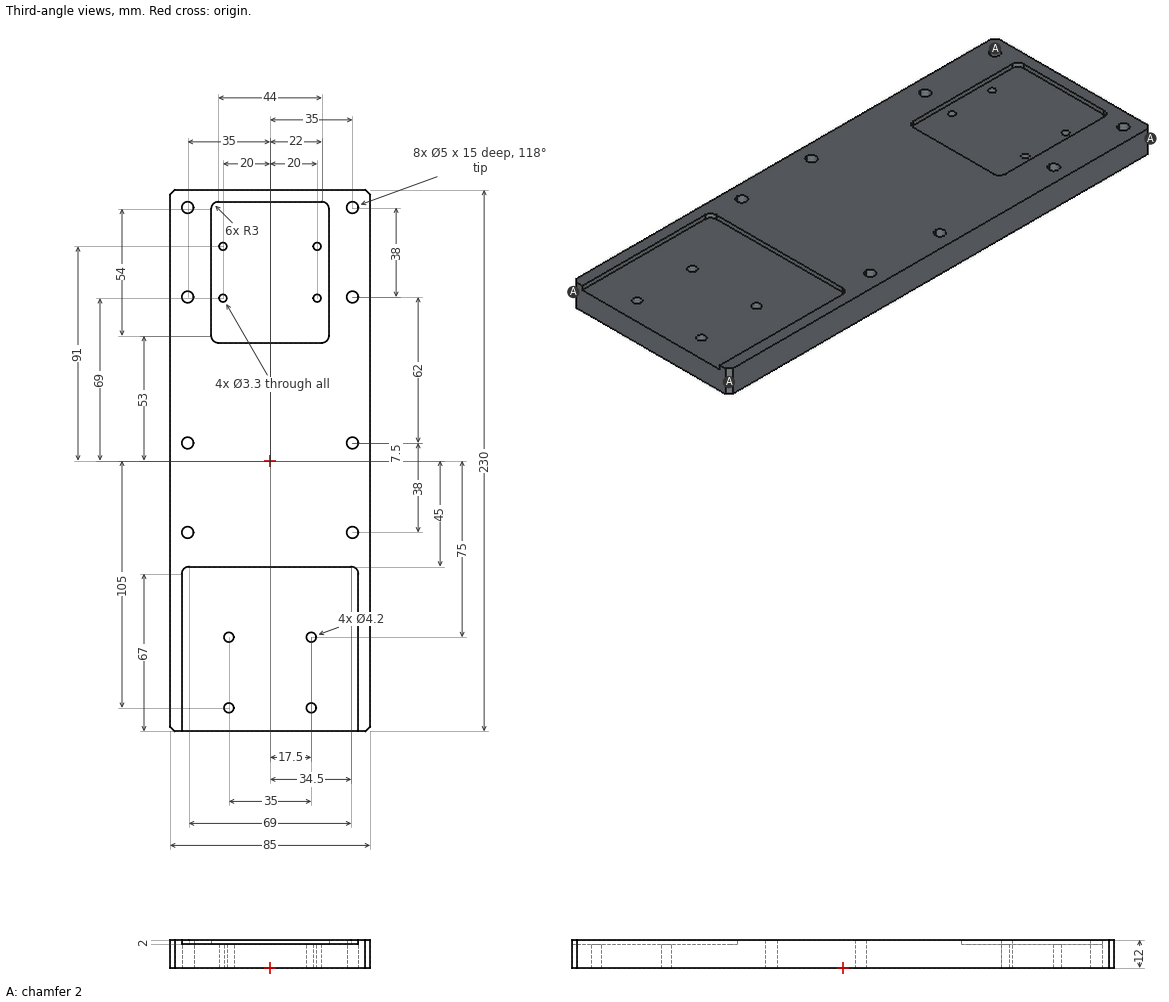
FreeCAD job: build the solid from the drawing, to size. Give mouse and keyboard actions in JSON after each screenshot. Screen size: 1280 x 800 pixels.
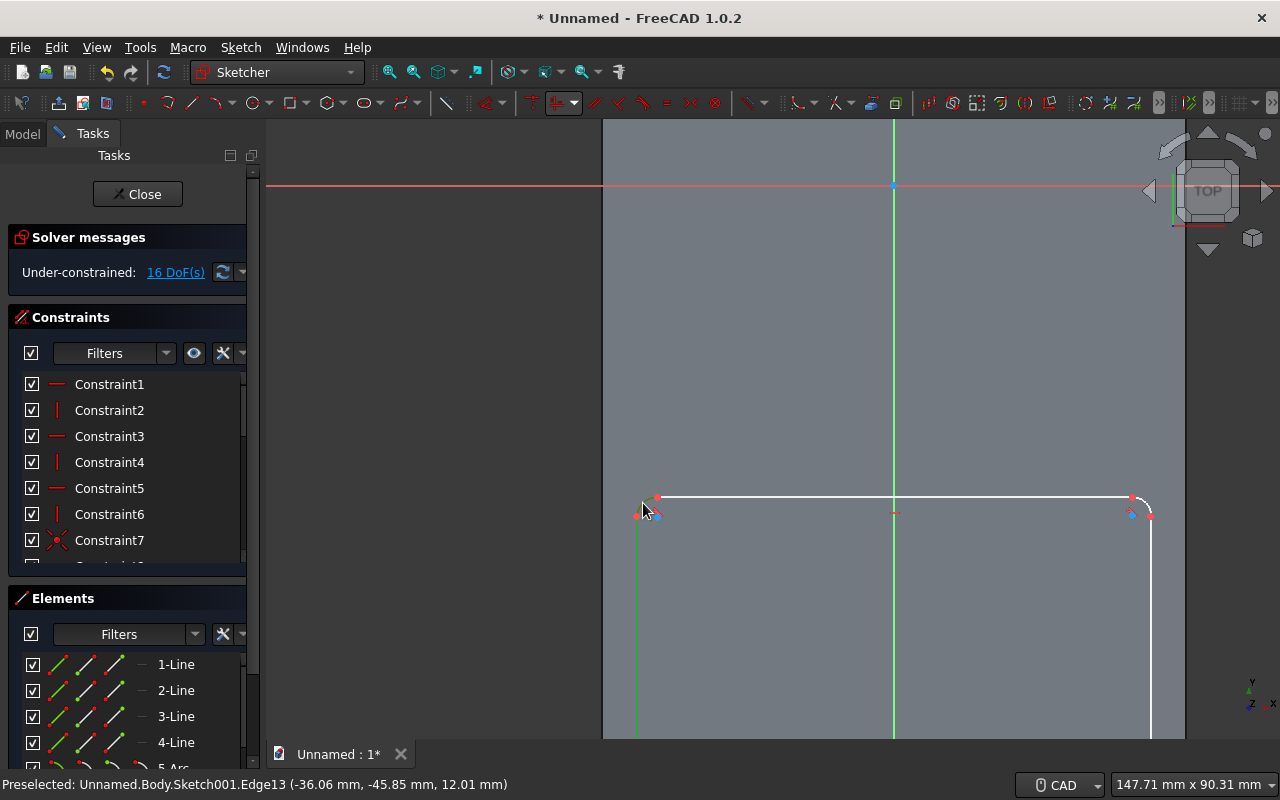
{"action": "key", "text": "t"}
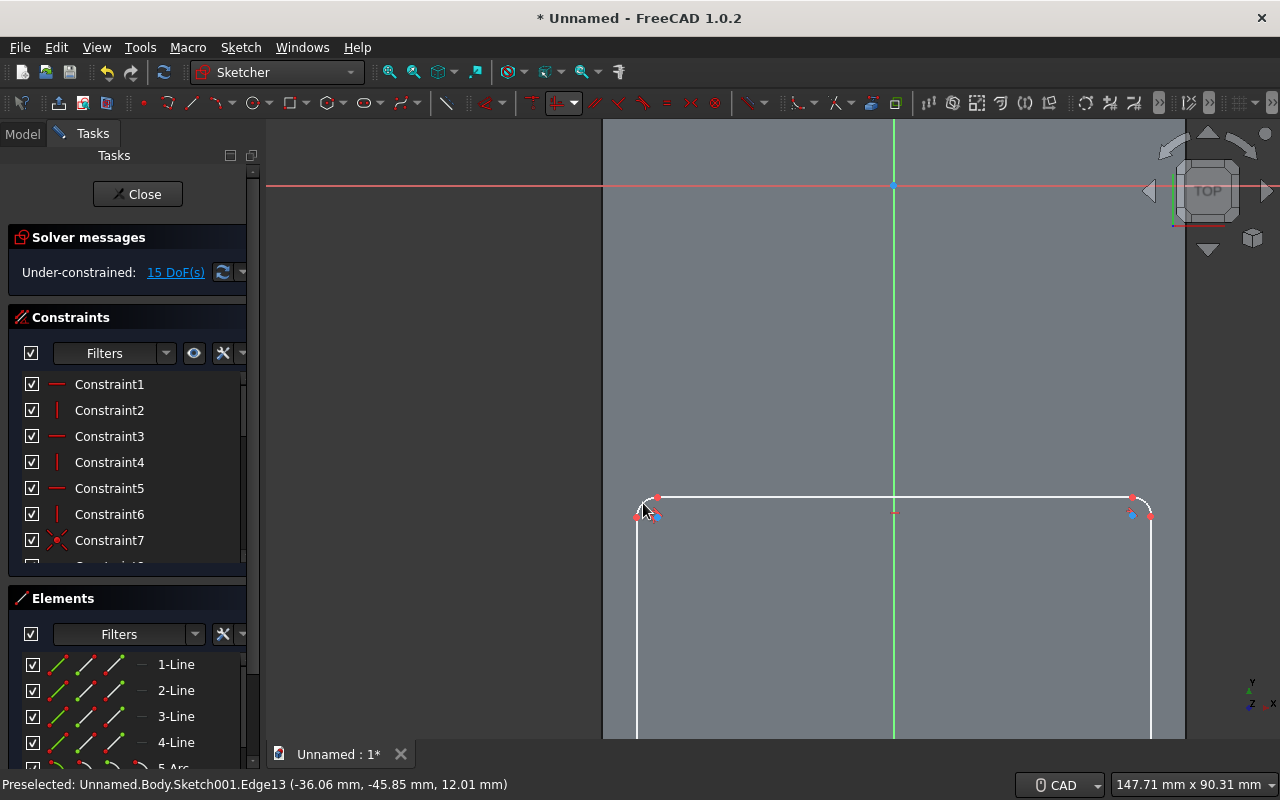
{"action": "scroll", "coordinate": [643, 503], "scroll_direction": "down", "scroll_amount": 7}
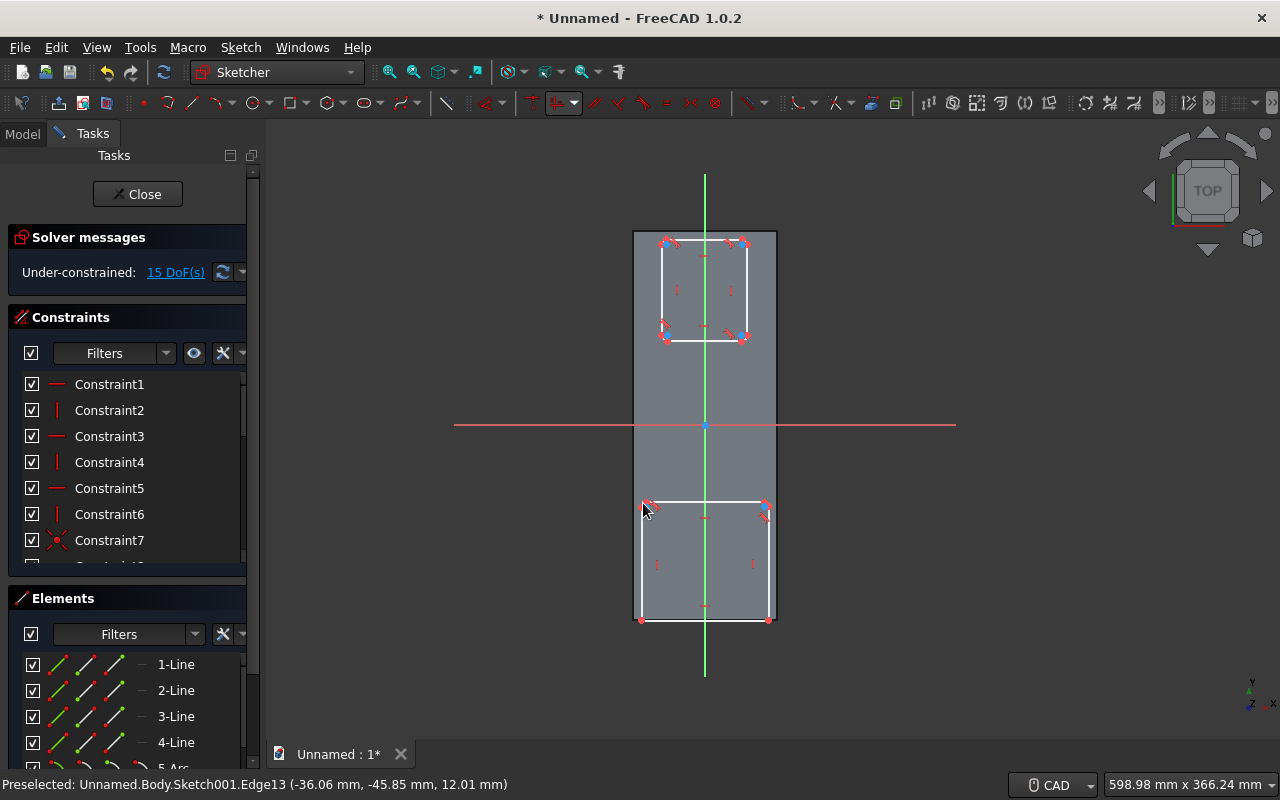
{"action": "left_click", "coordinate": [769, 587]}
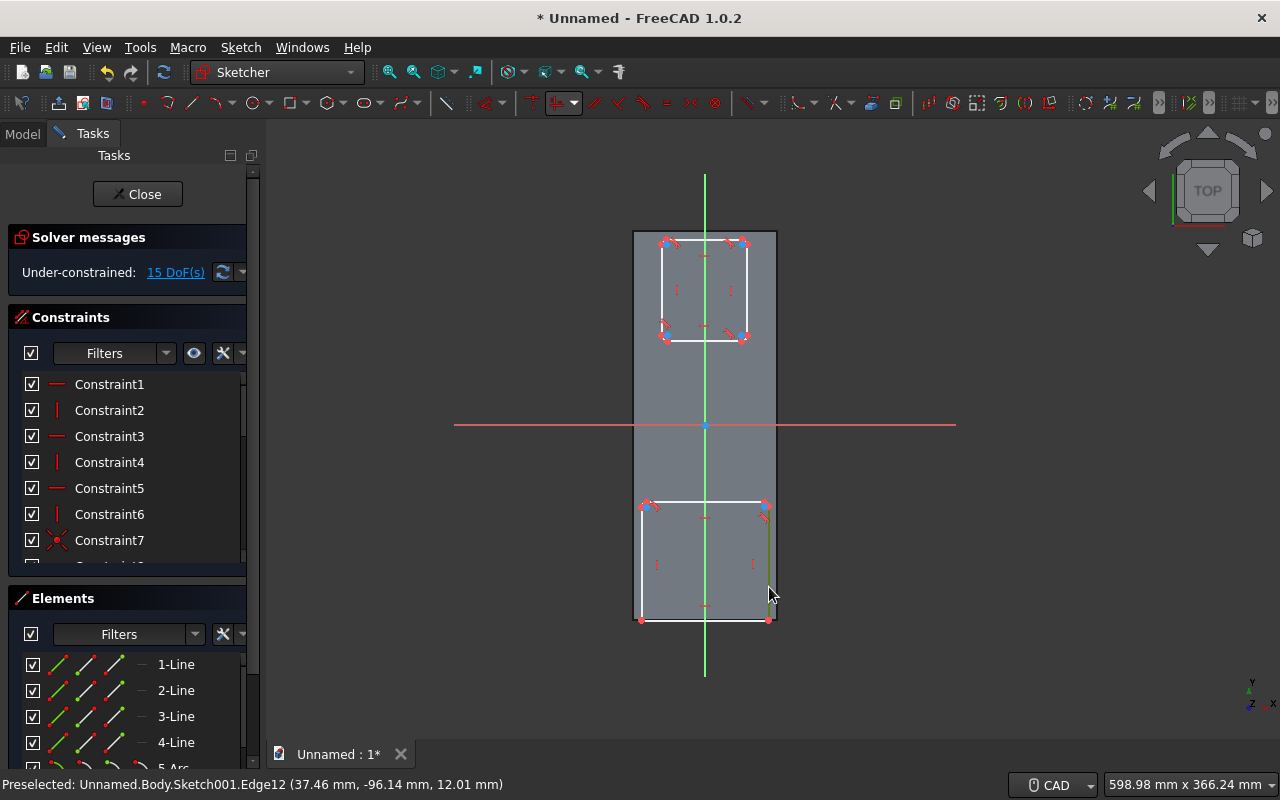
{"action": "scroll", "coordinate": [767, 503], "scroll_direction": "up", "scroll_amount": 7}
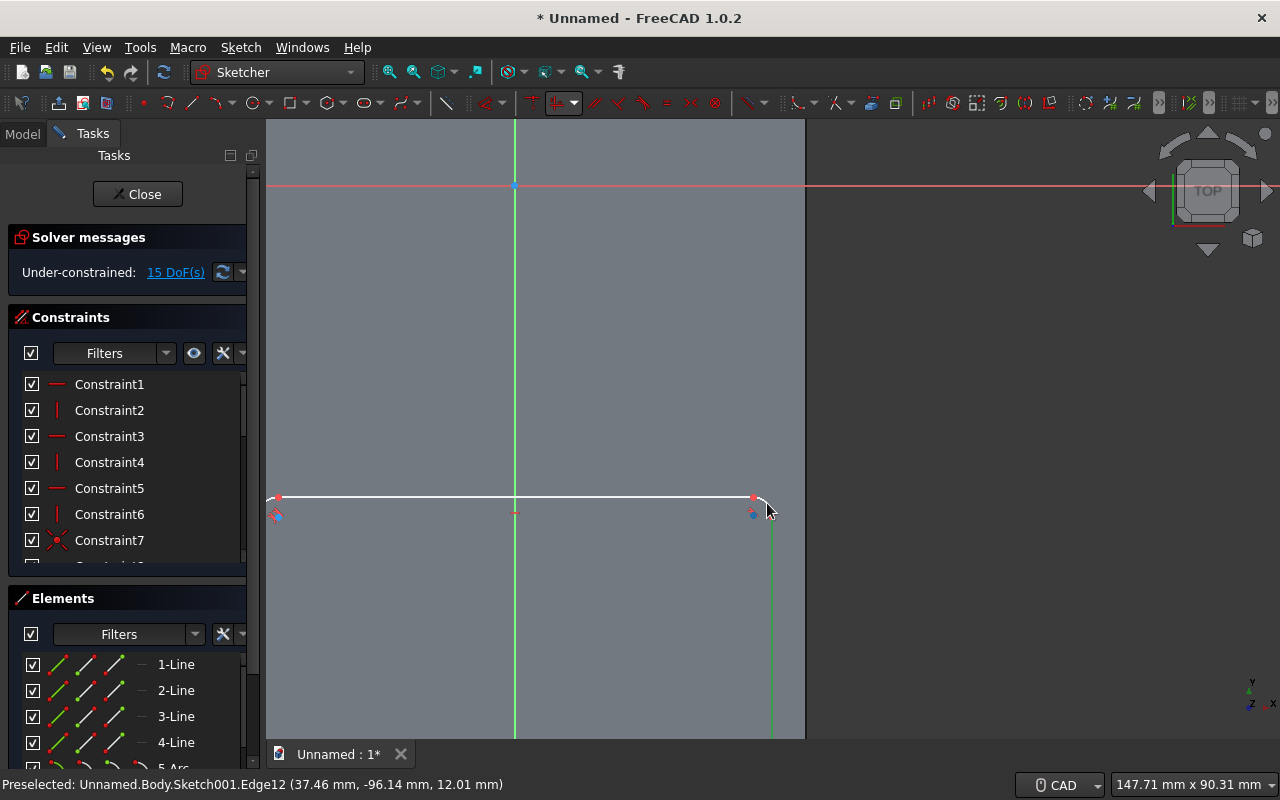
{"action": "left_click", "coordinate": [767, 503]}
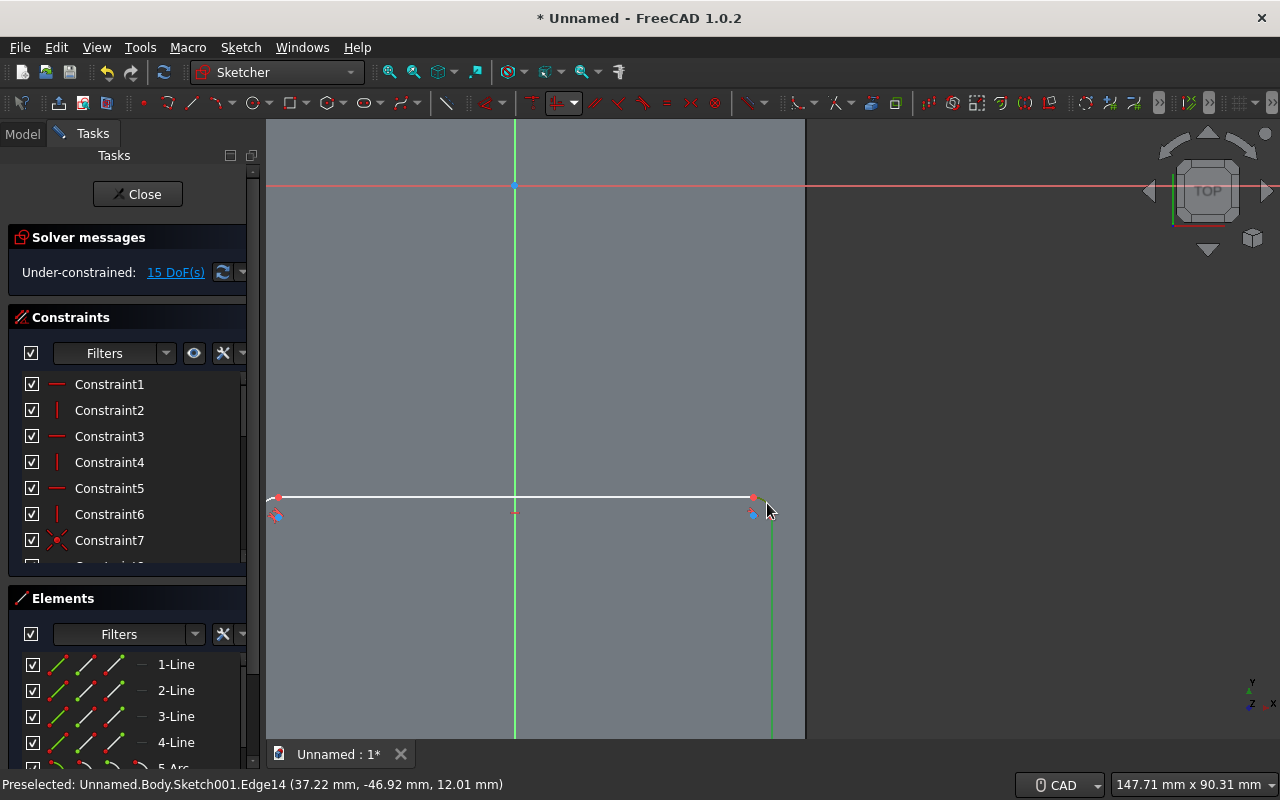
{"action": "key", "text": "t"}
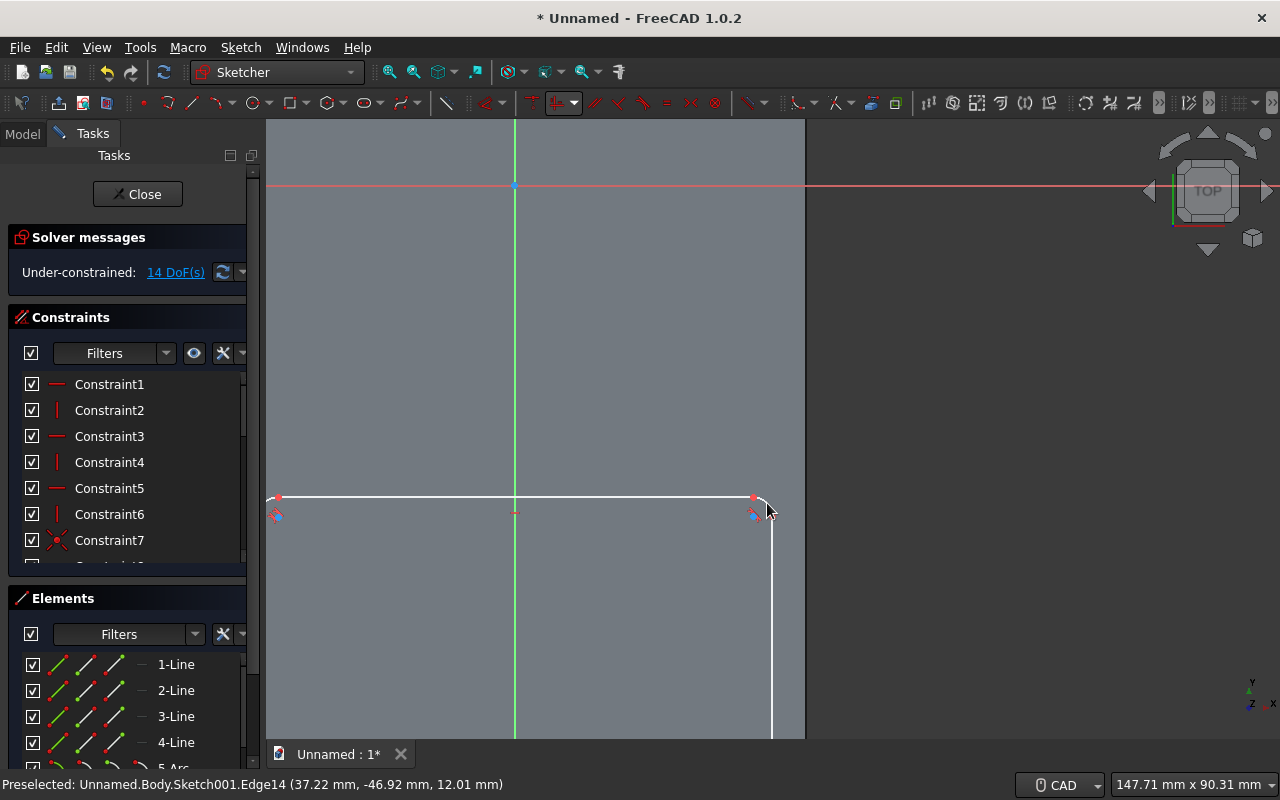
{"action": "scroll", "coordinate": [767, 503], "scroll_direction": "down", "scroll_amount": 7}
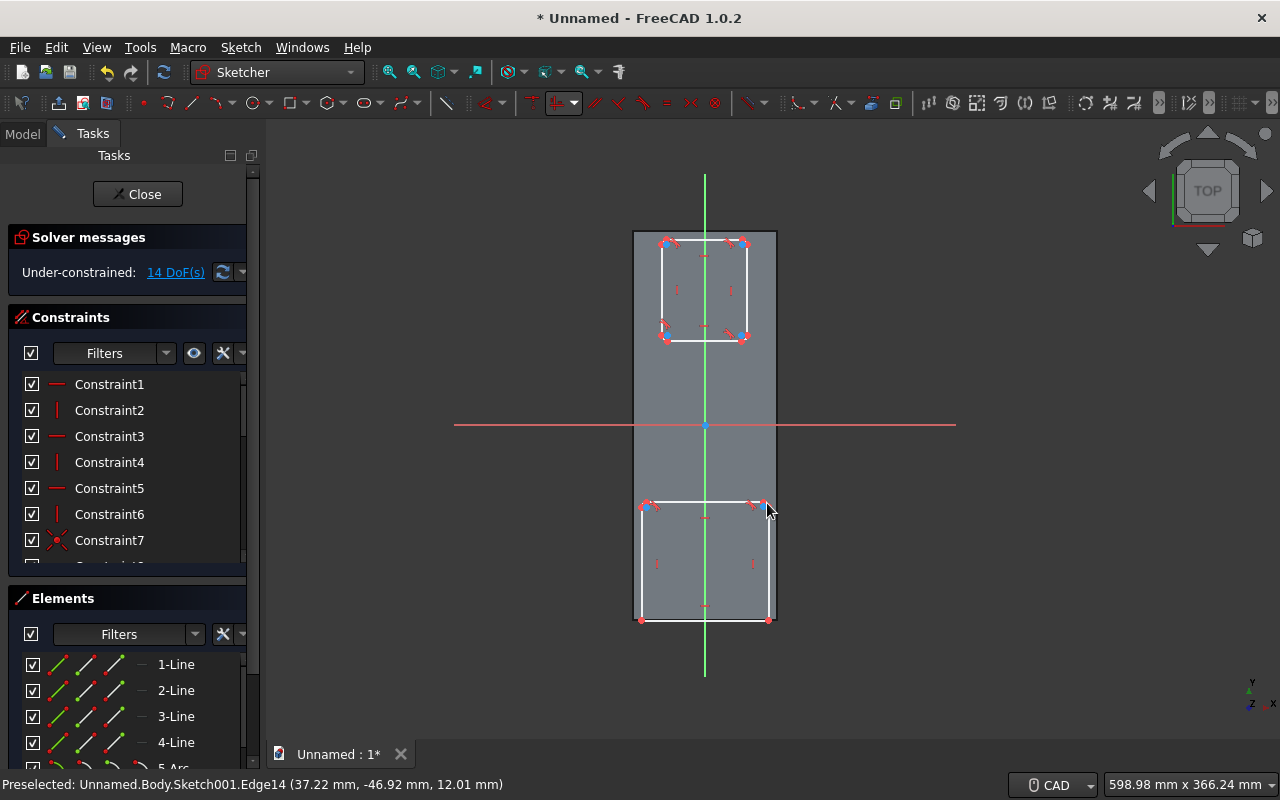
{"action": "scroll", "coordinate": [664, 240], "scroll_direction": "up", "scroll_amount": 9}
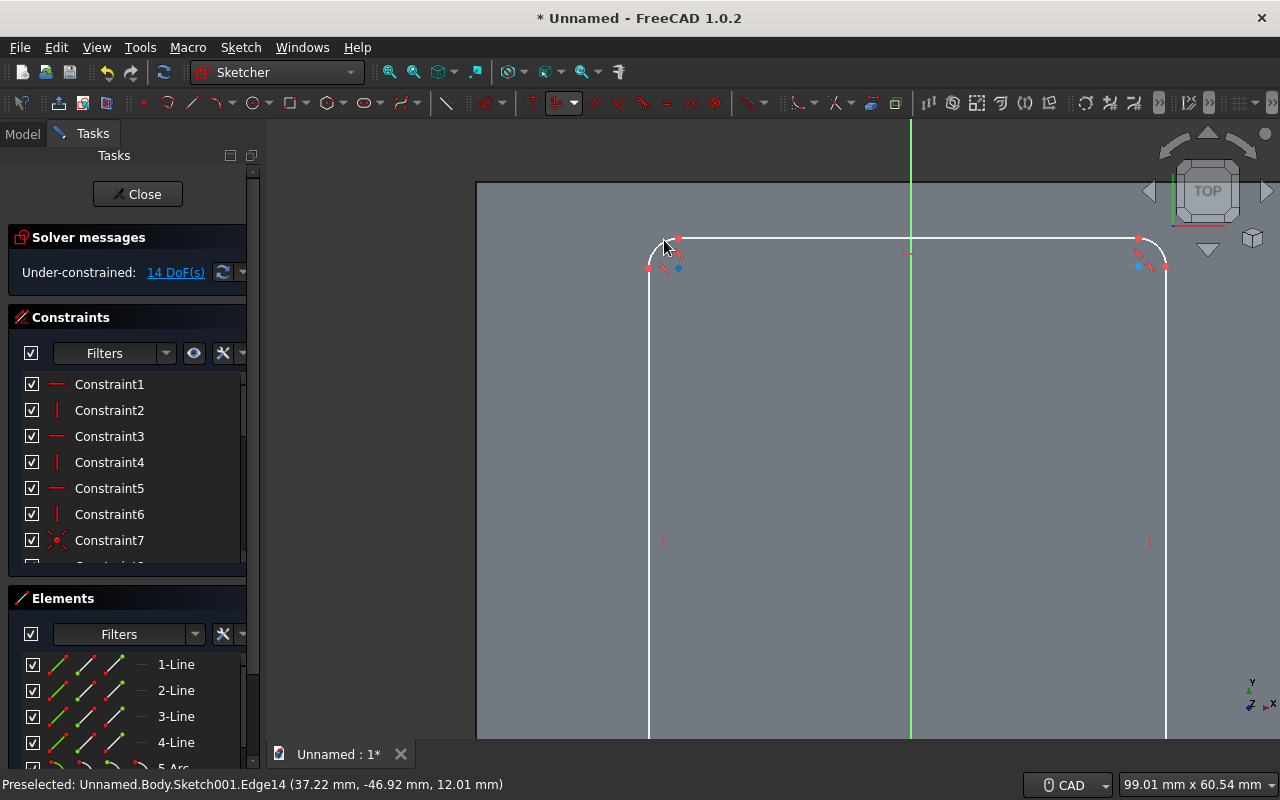
{"action": "left_click", "coordinate": [665, 242]}